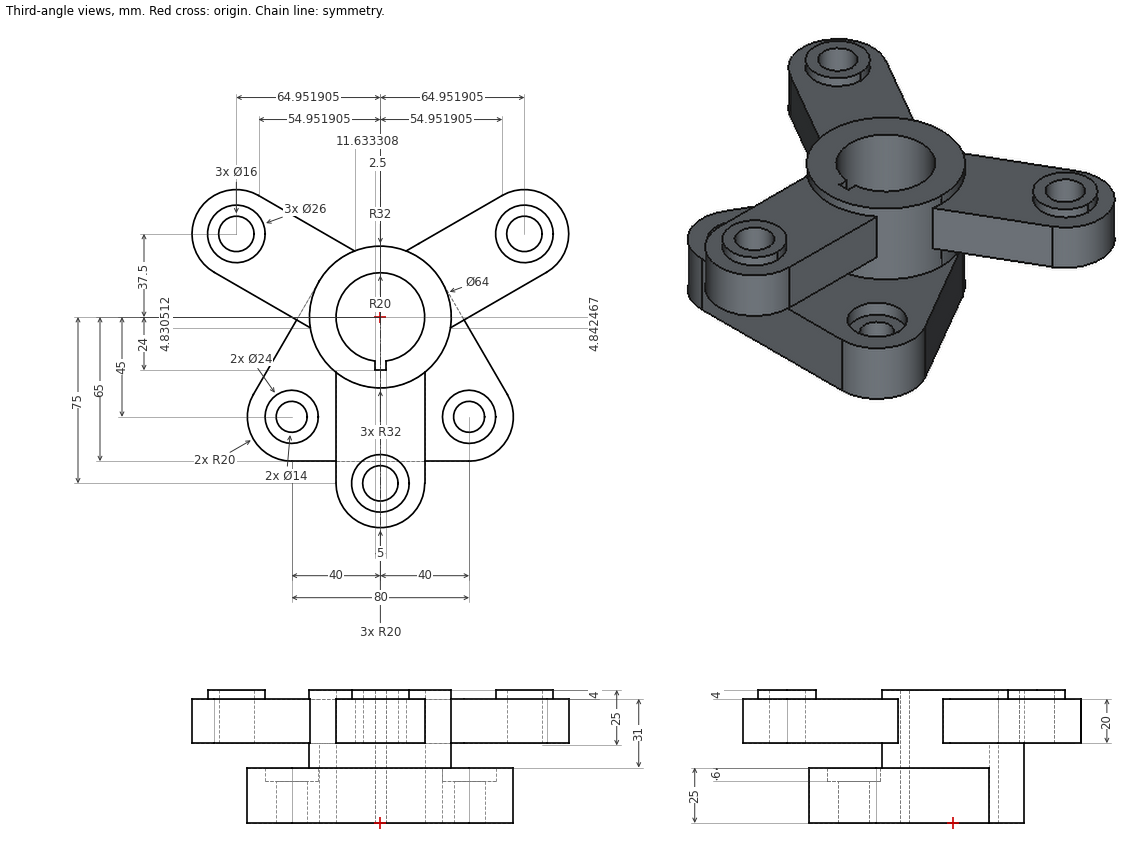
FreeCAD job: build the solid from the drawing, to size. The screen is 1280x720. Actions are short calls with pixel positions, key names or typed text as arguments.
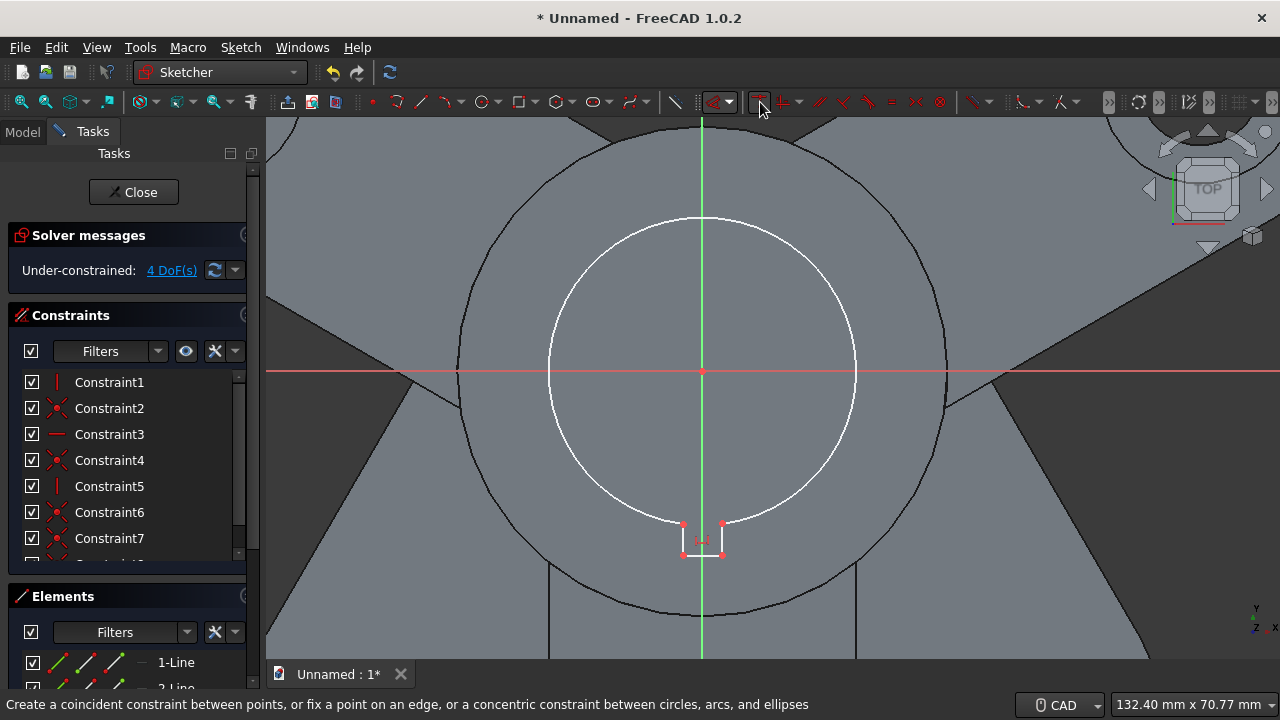
click(846, 316)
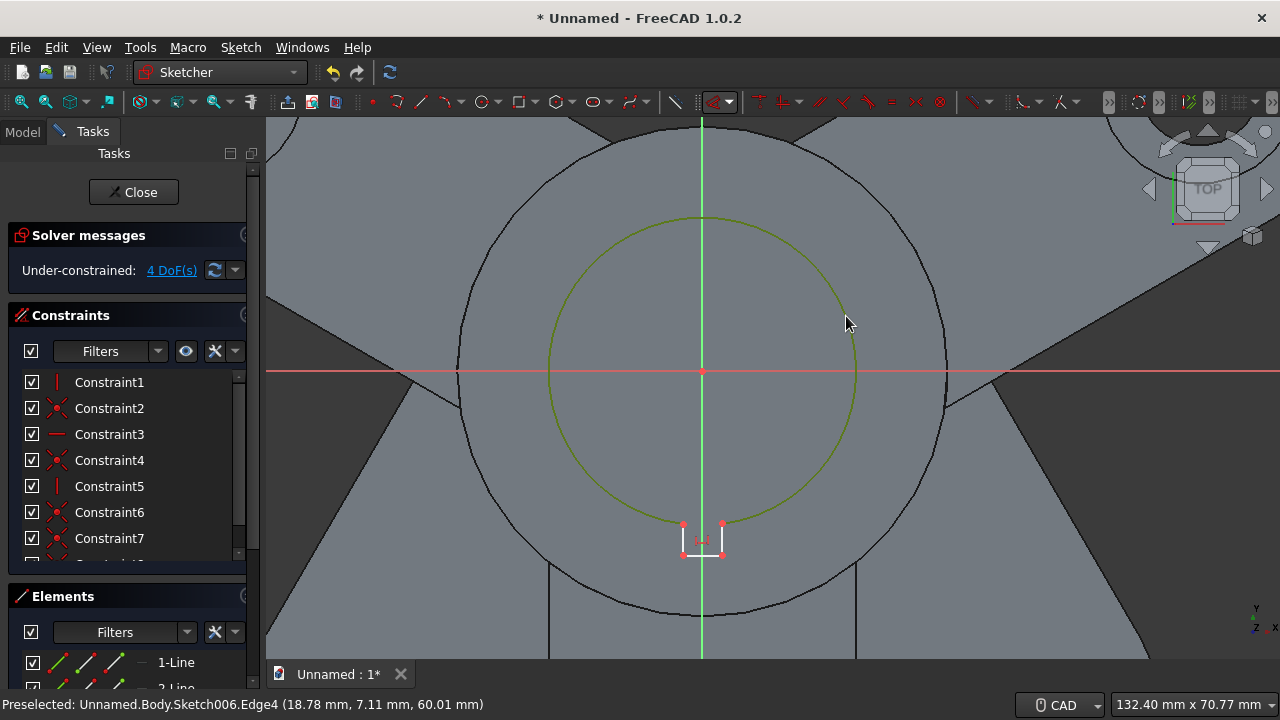
key(k)
key(r)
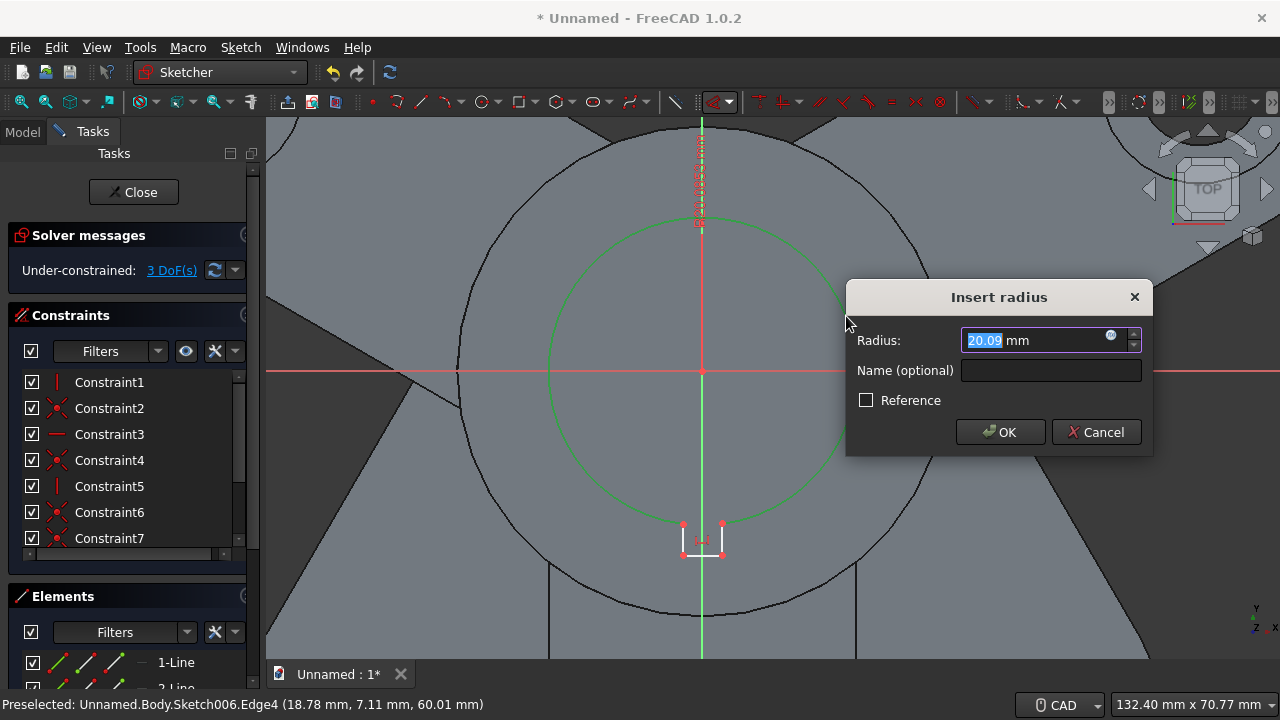
text(20)
key(Return)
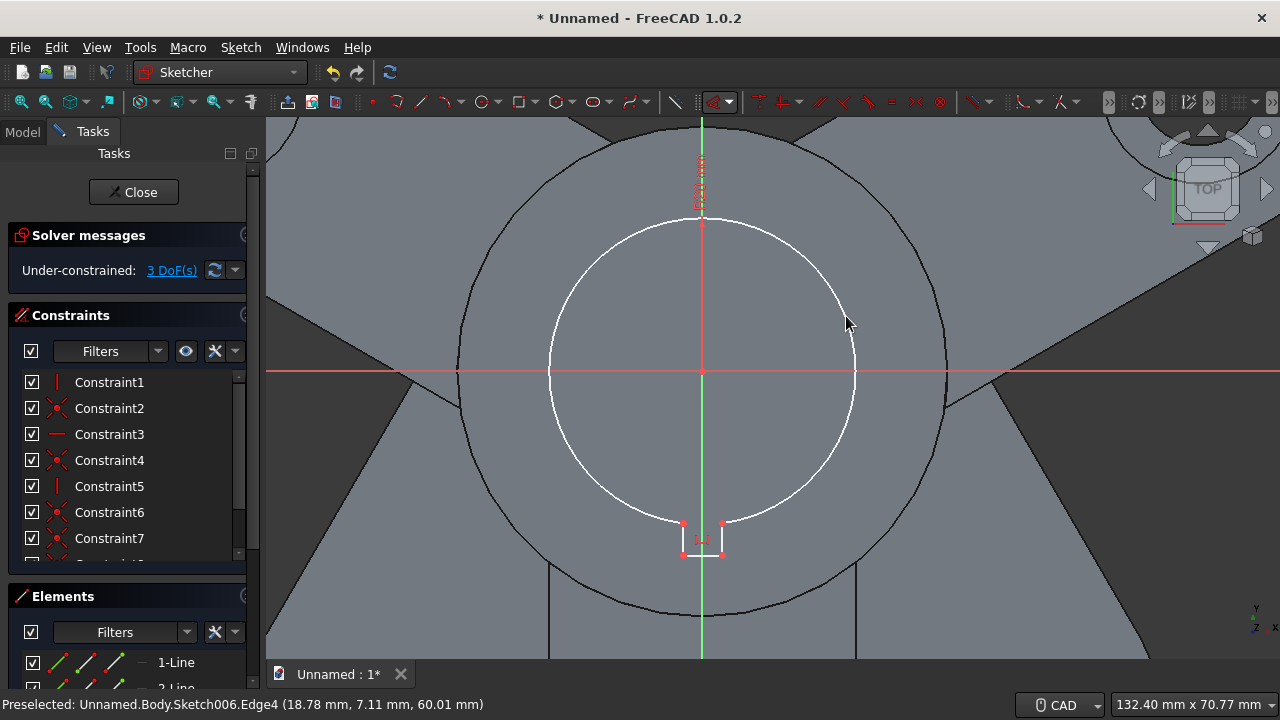
click(699, 556)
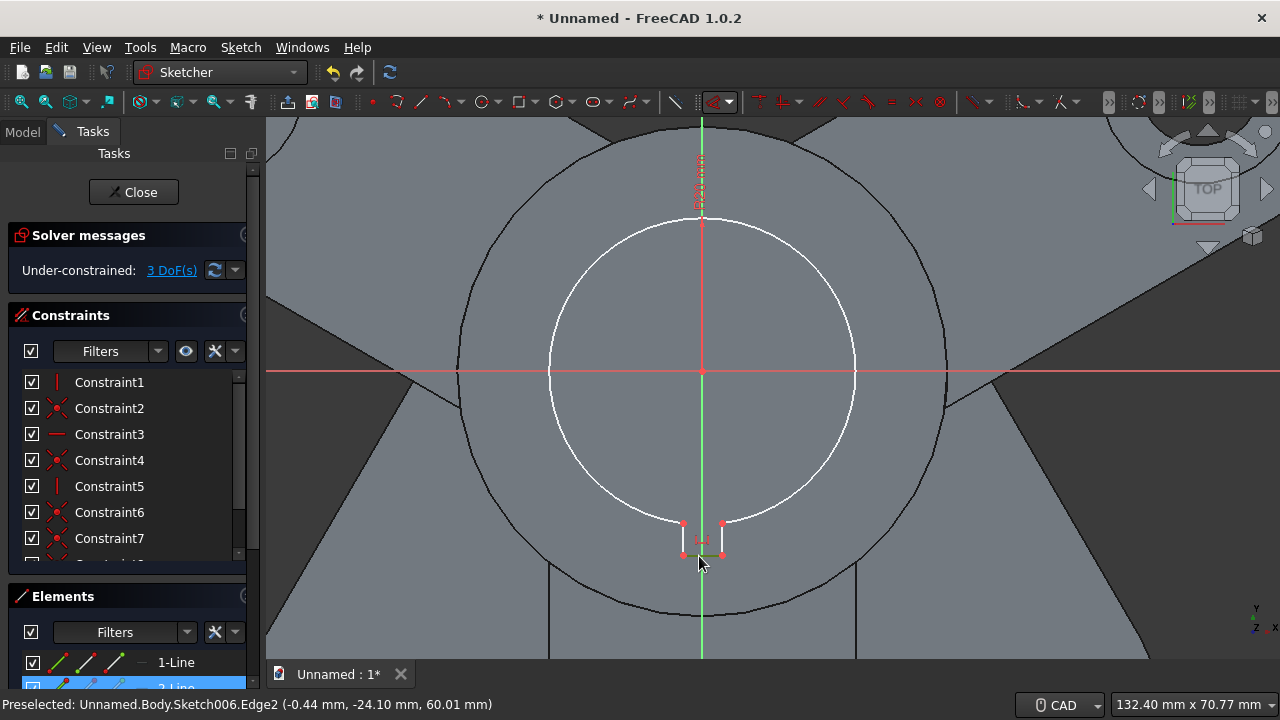
key(l)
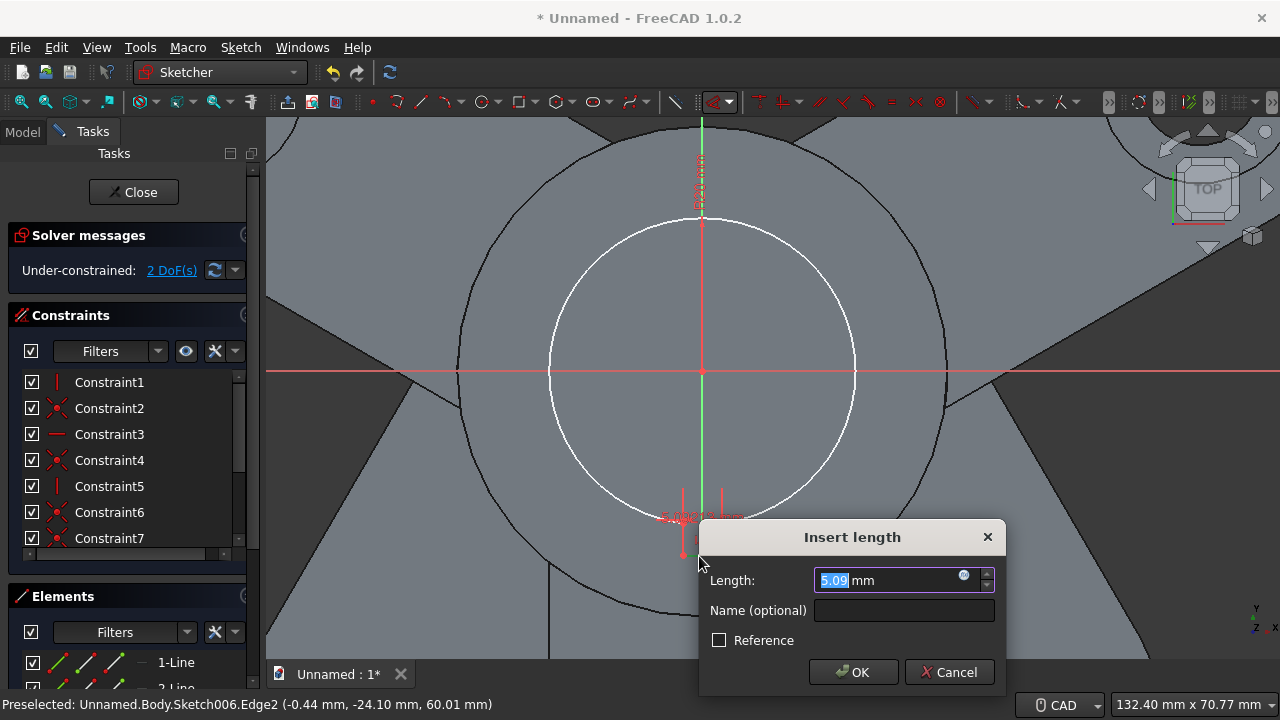
text(5)
key(Return)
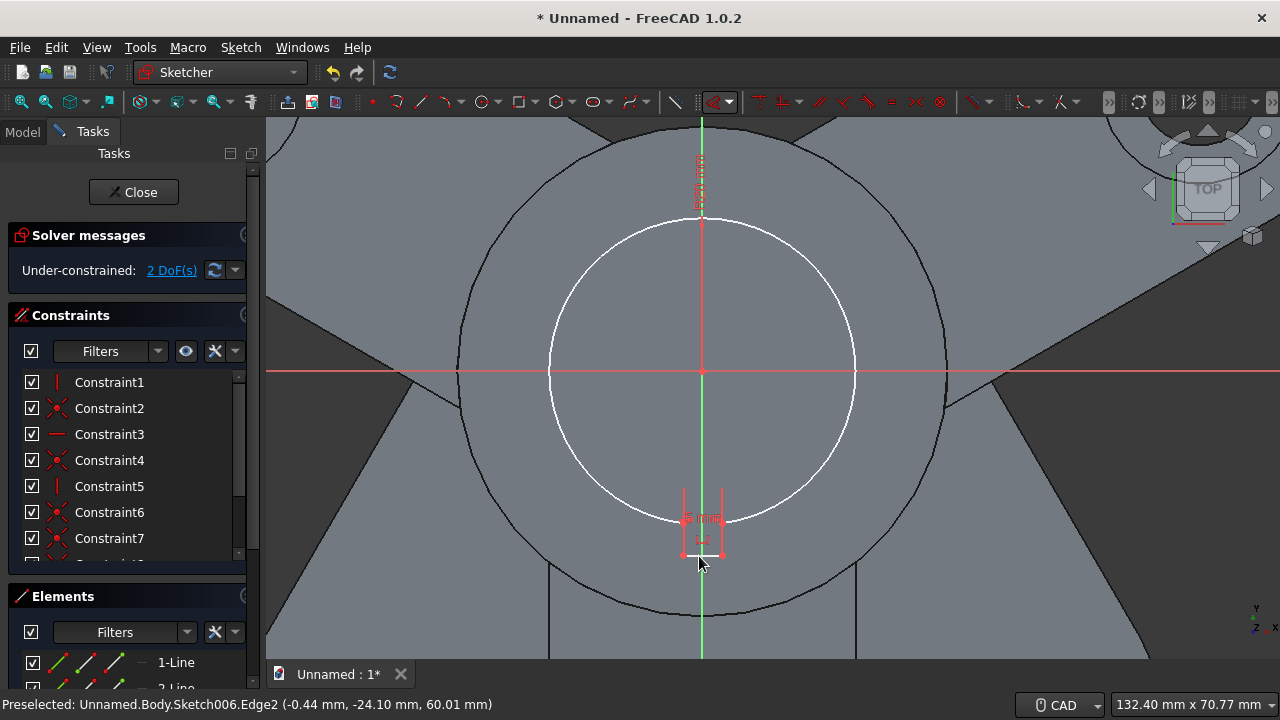
click(684, 556)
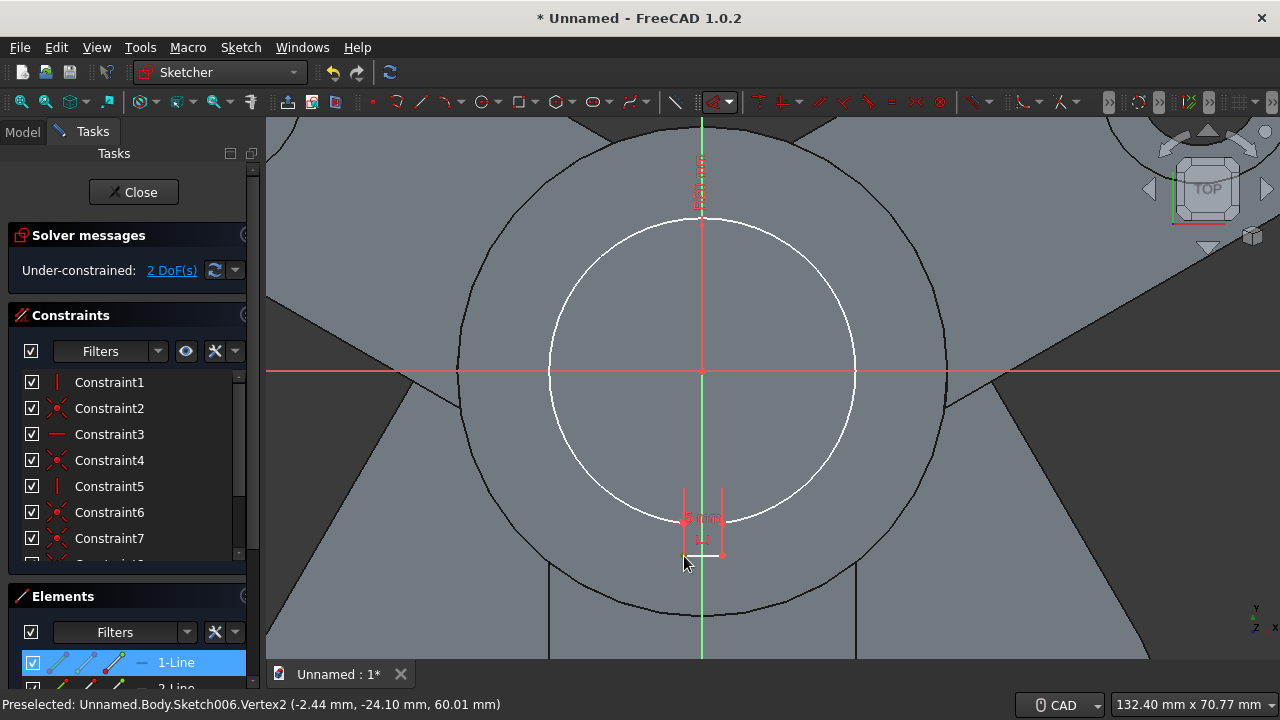
key(i)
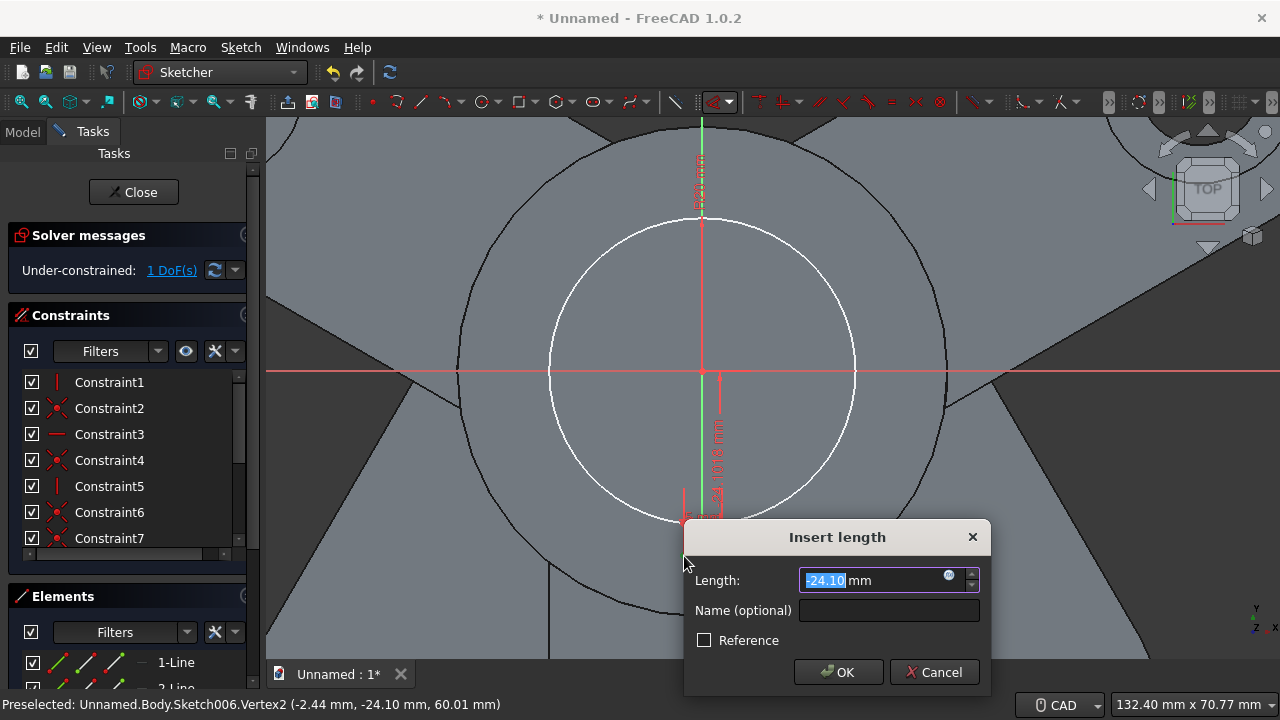
text(-24)
key(Return)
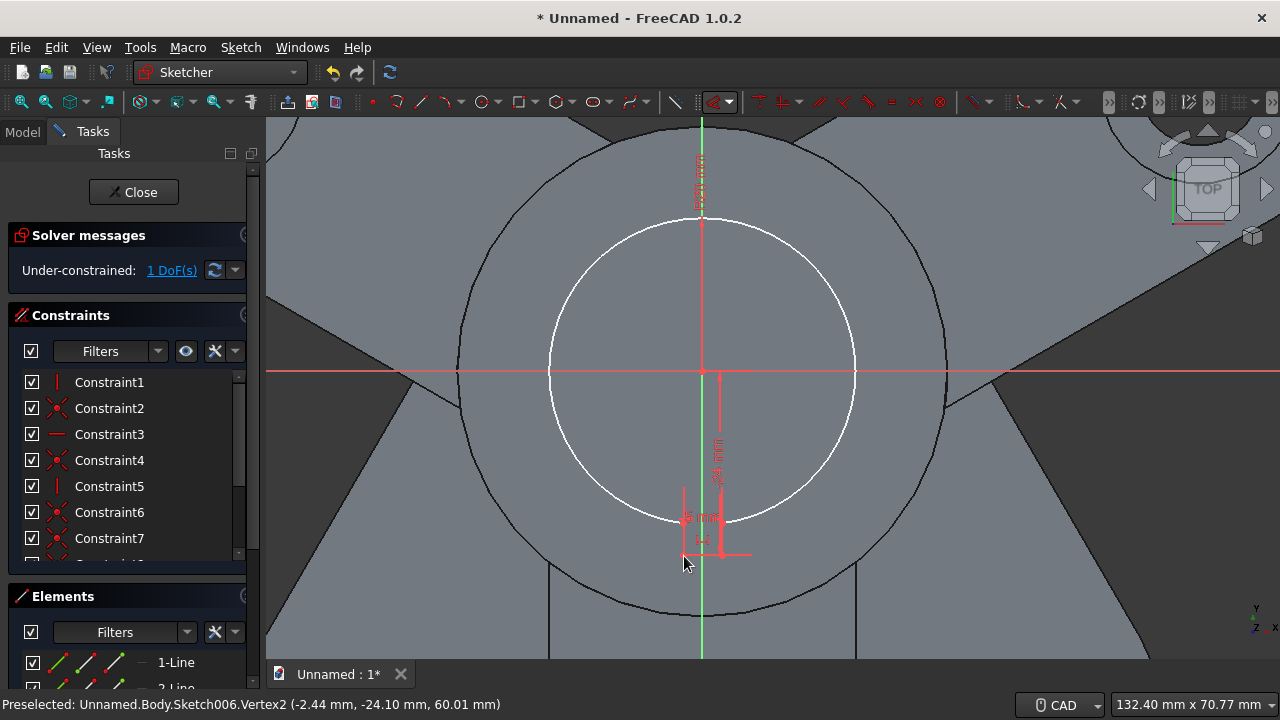
scroll(684, 523, up, 4)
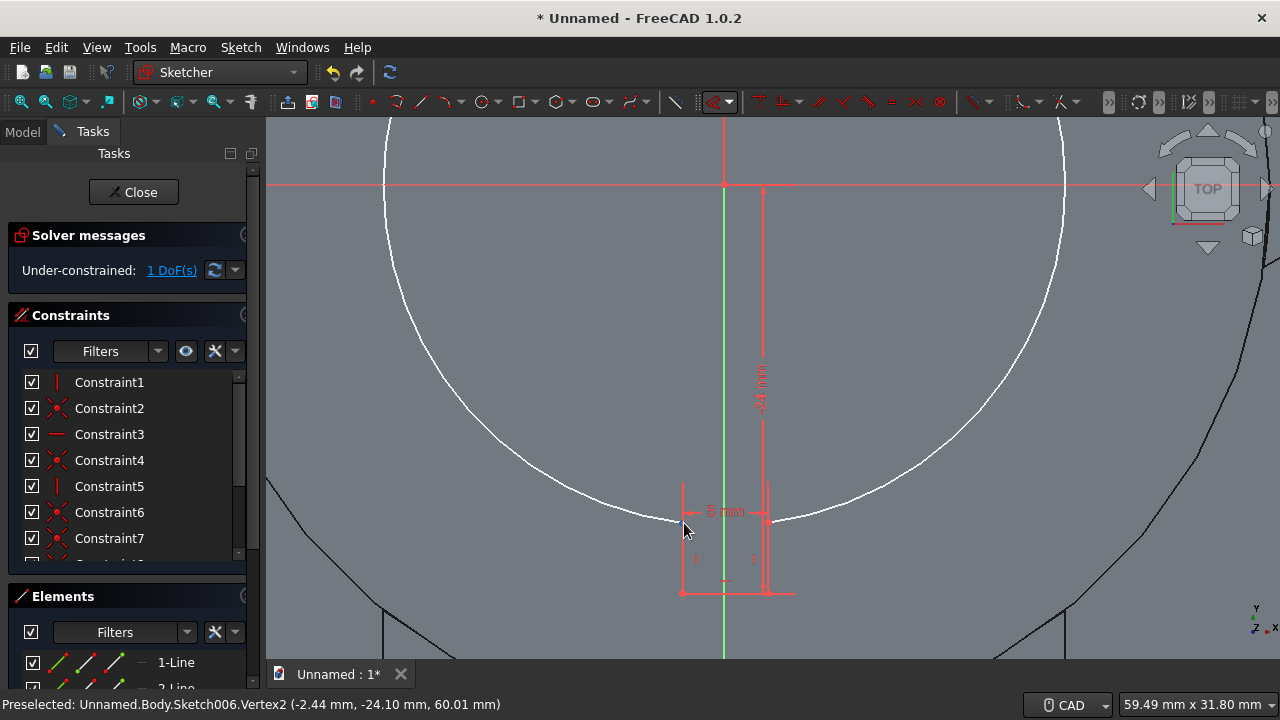
click(683, 523)